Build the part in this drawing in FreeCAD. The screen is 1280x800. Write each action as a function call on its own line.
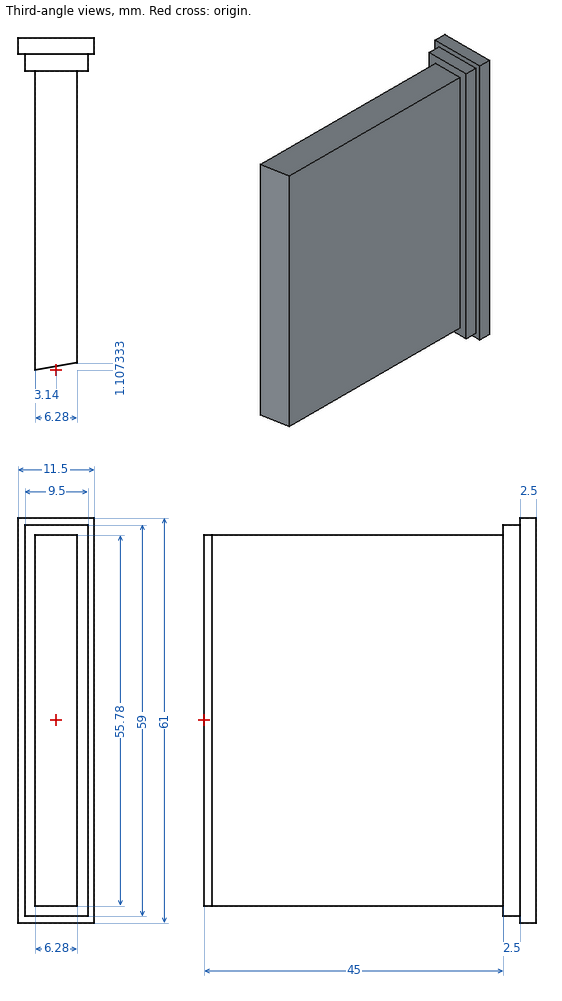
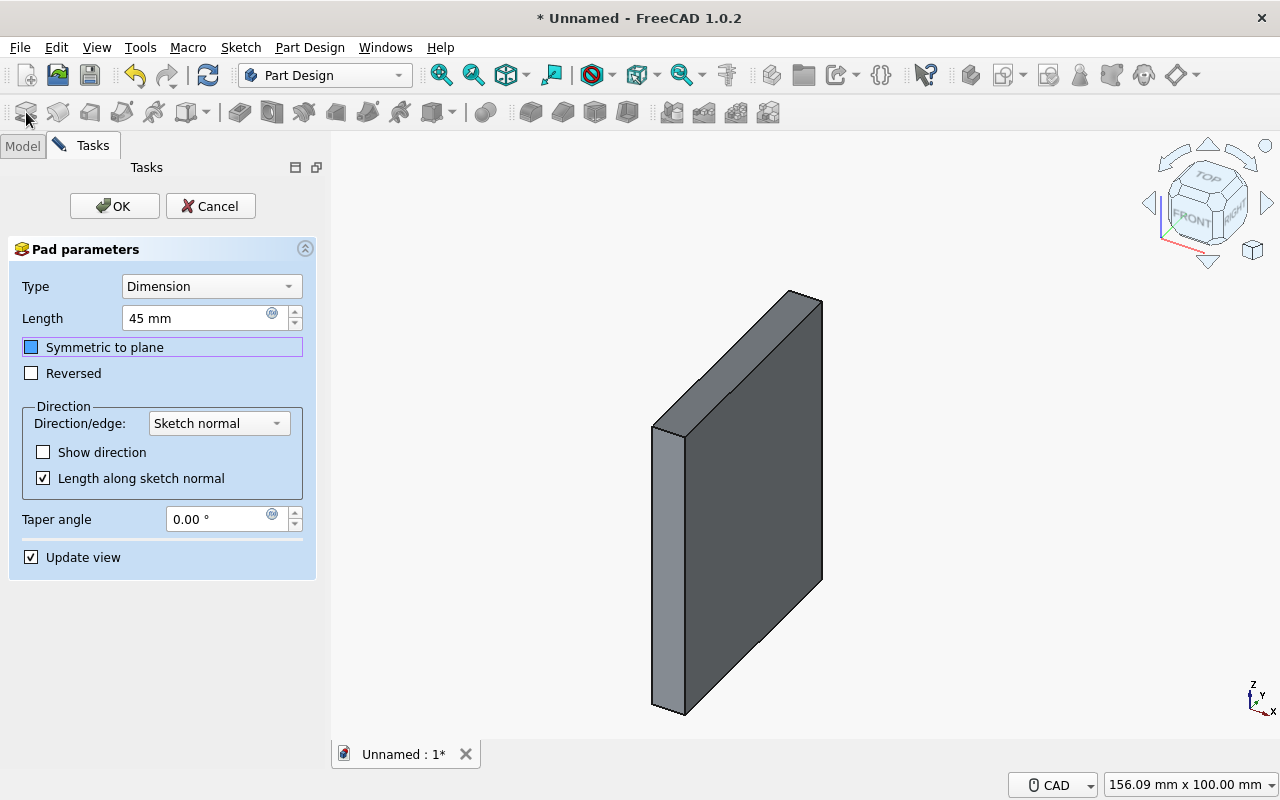
click(30, 373)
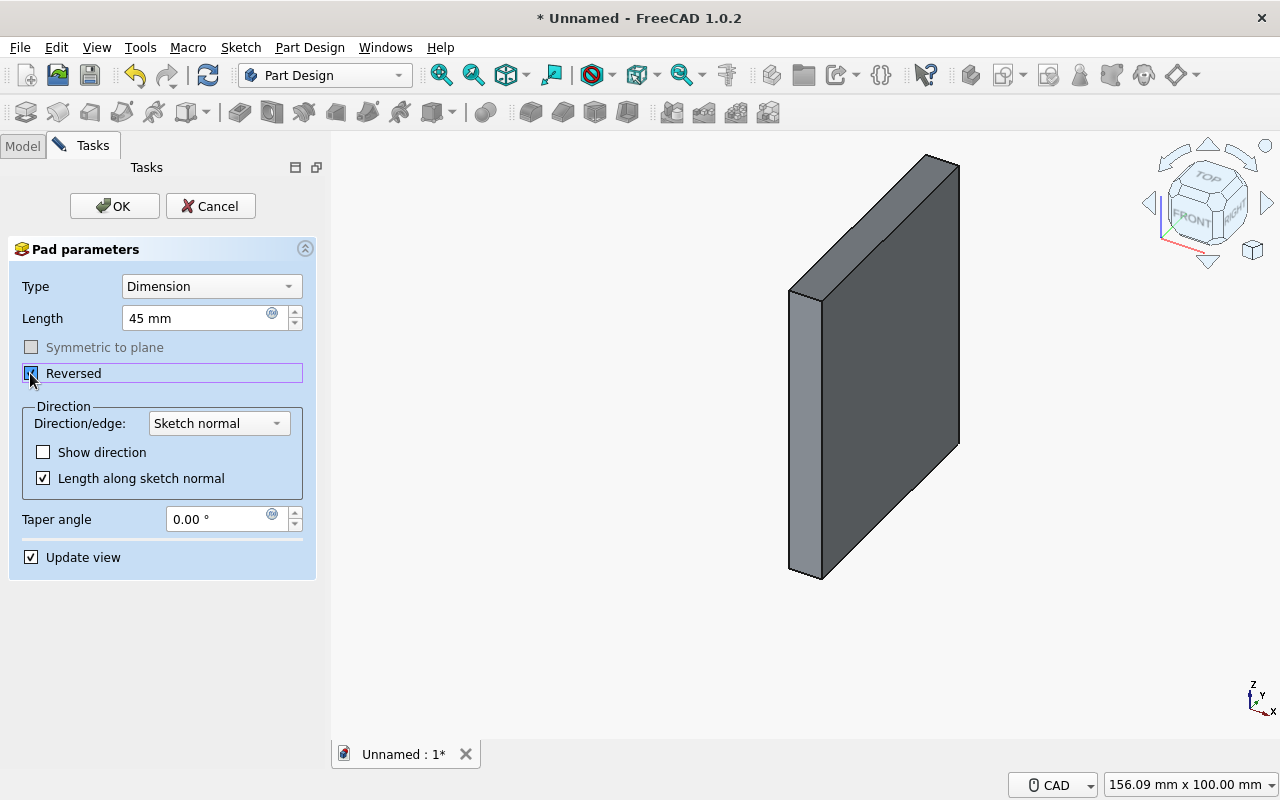
click(115, 206)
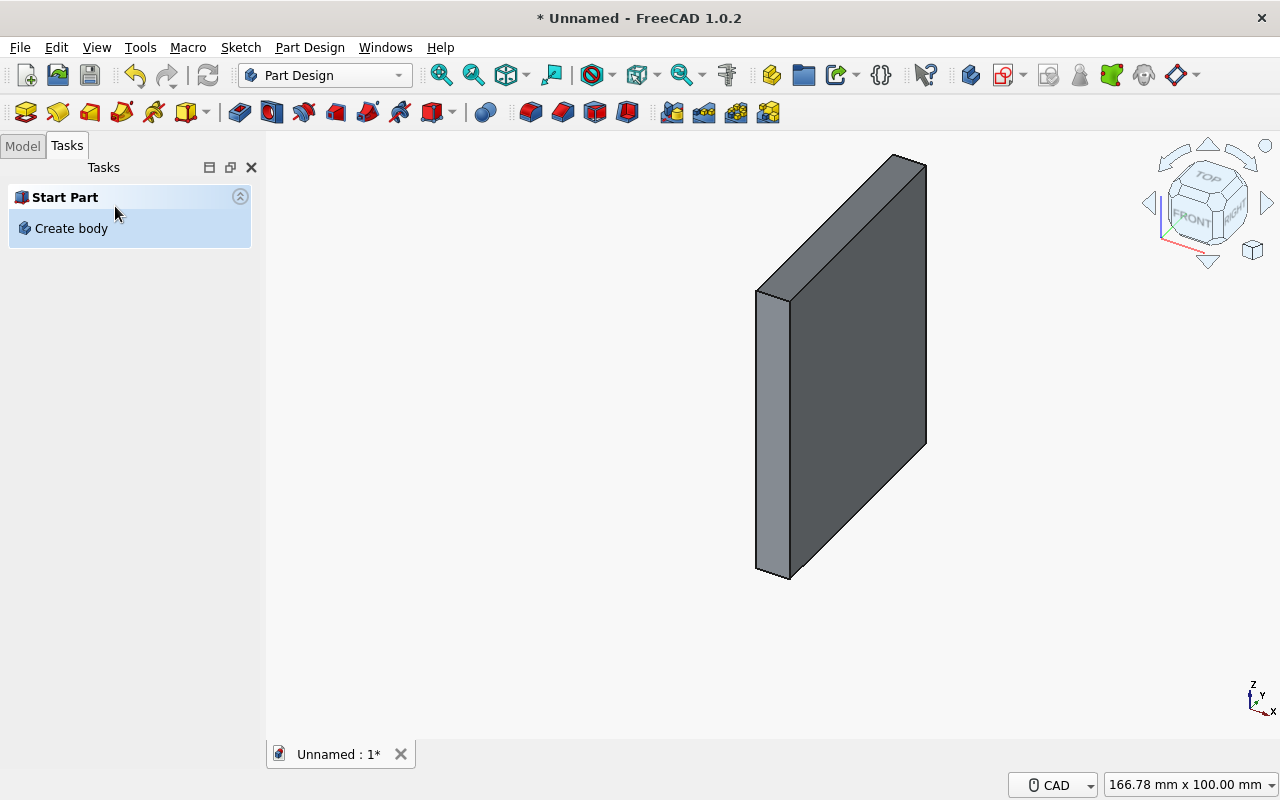
click(900, 169)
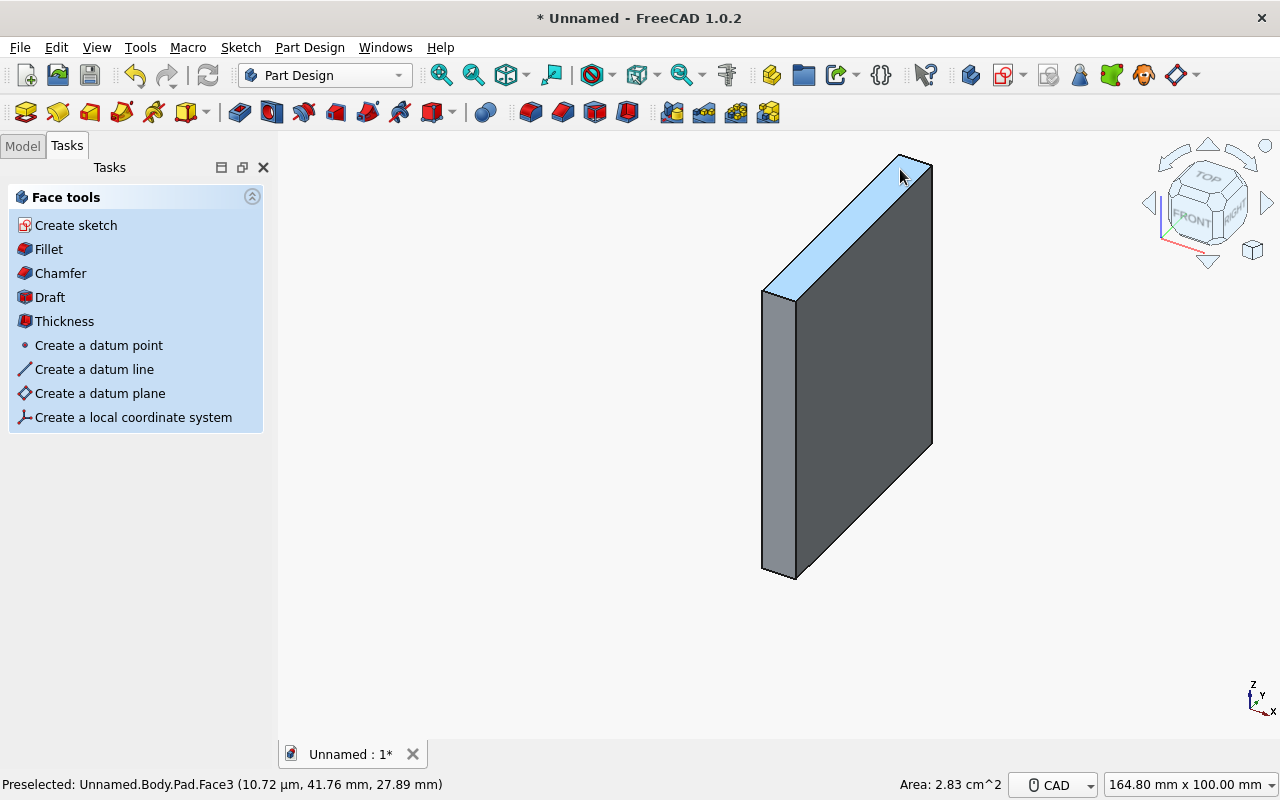
click(1004, 76)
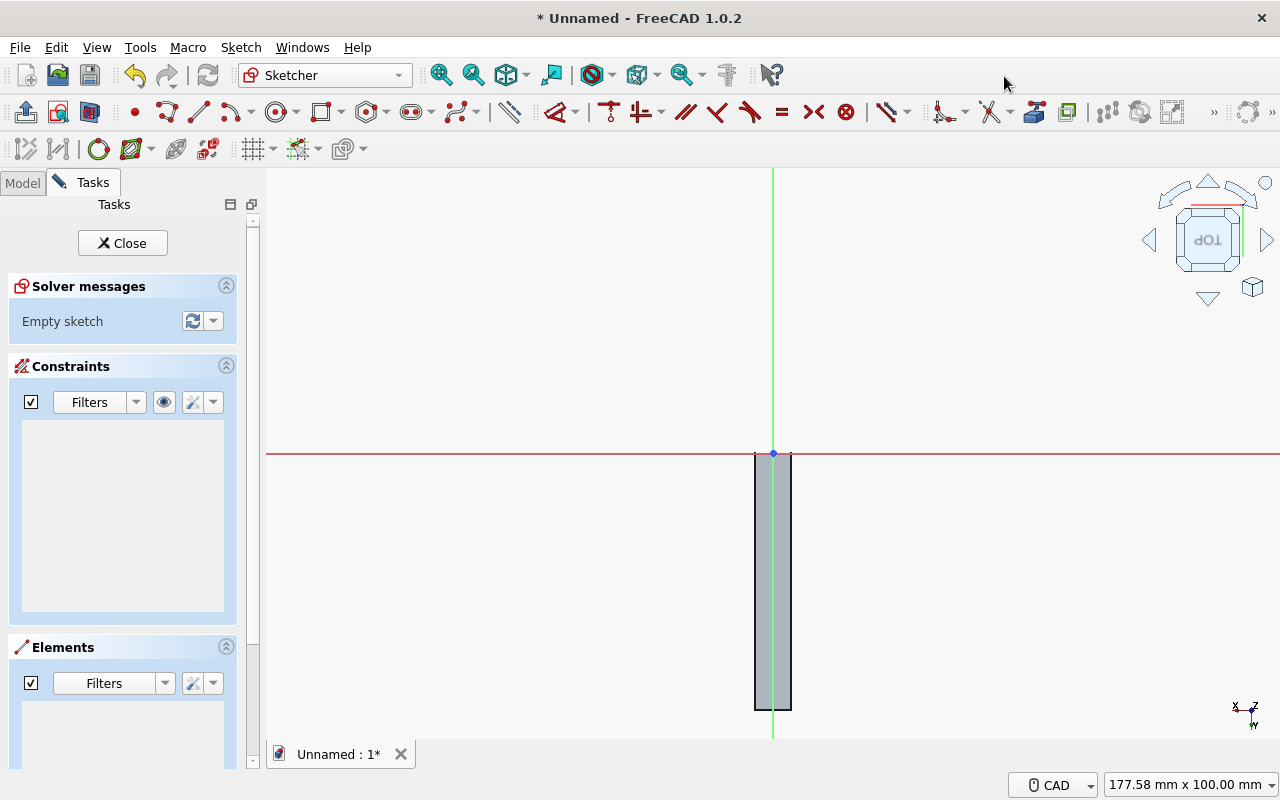
scroll(777, 457, up, 14)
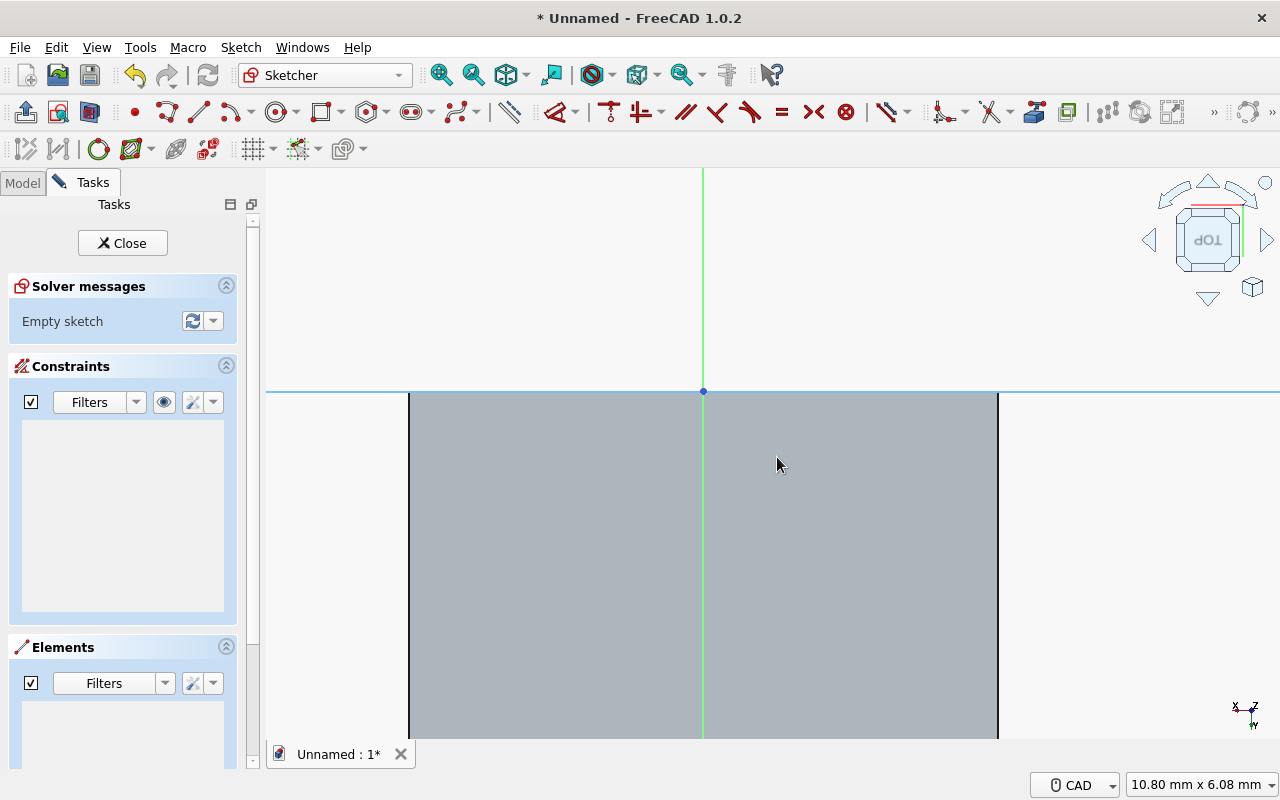
click(168, 112)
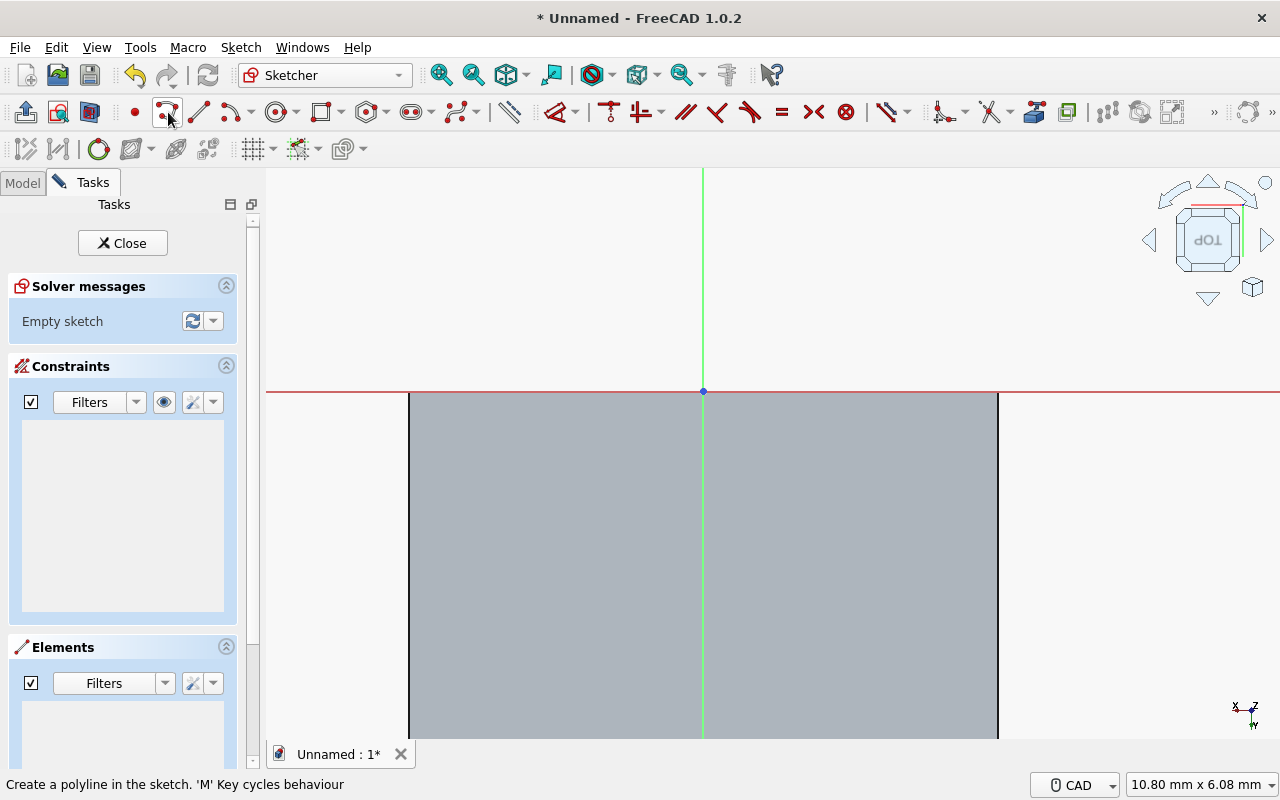
click(998, 392)
click(409, 401)
click(409, 496)
click(998, 392)
key(Escape)
key(Escape)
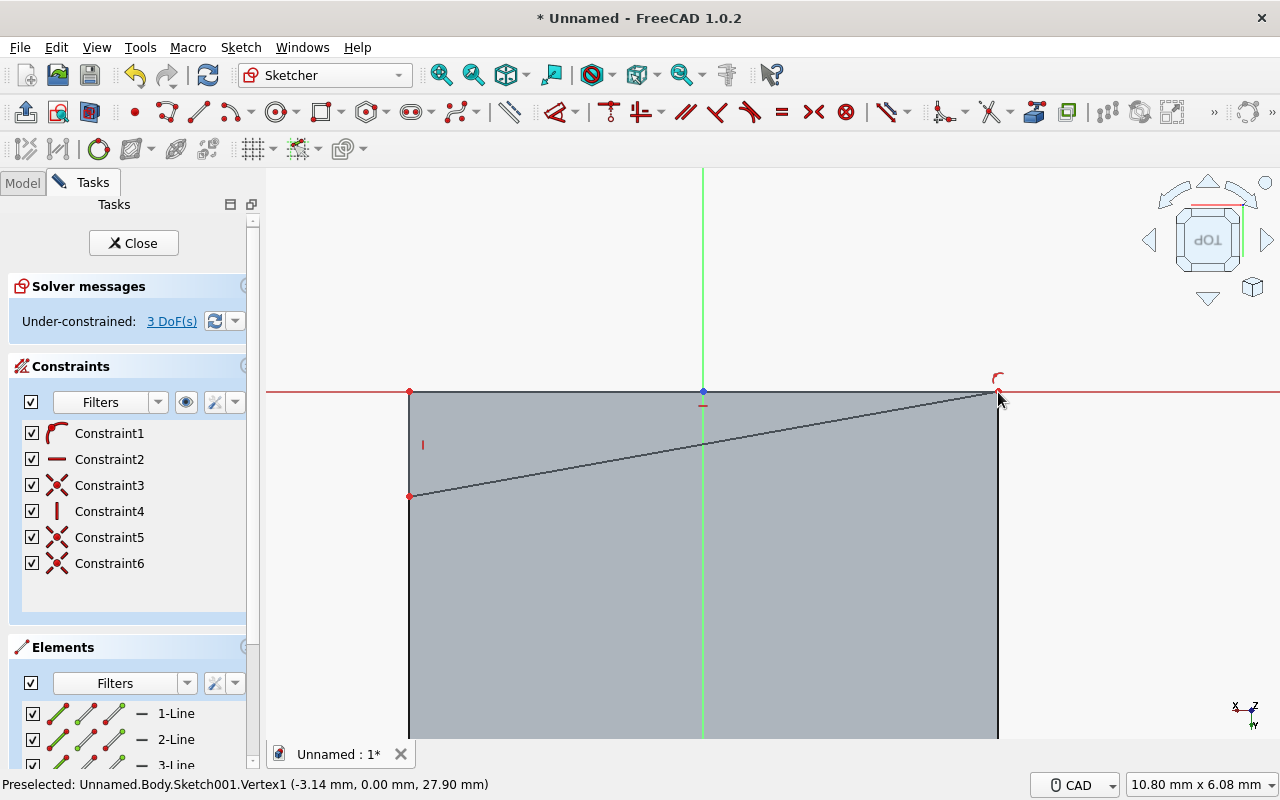
click(556, 112)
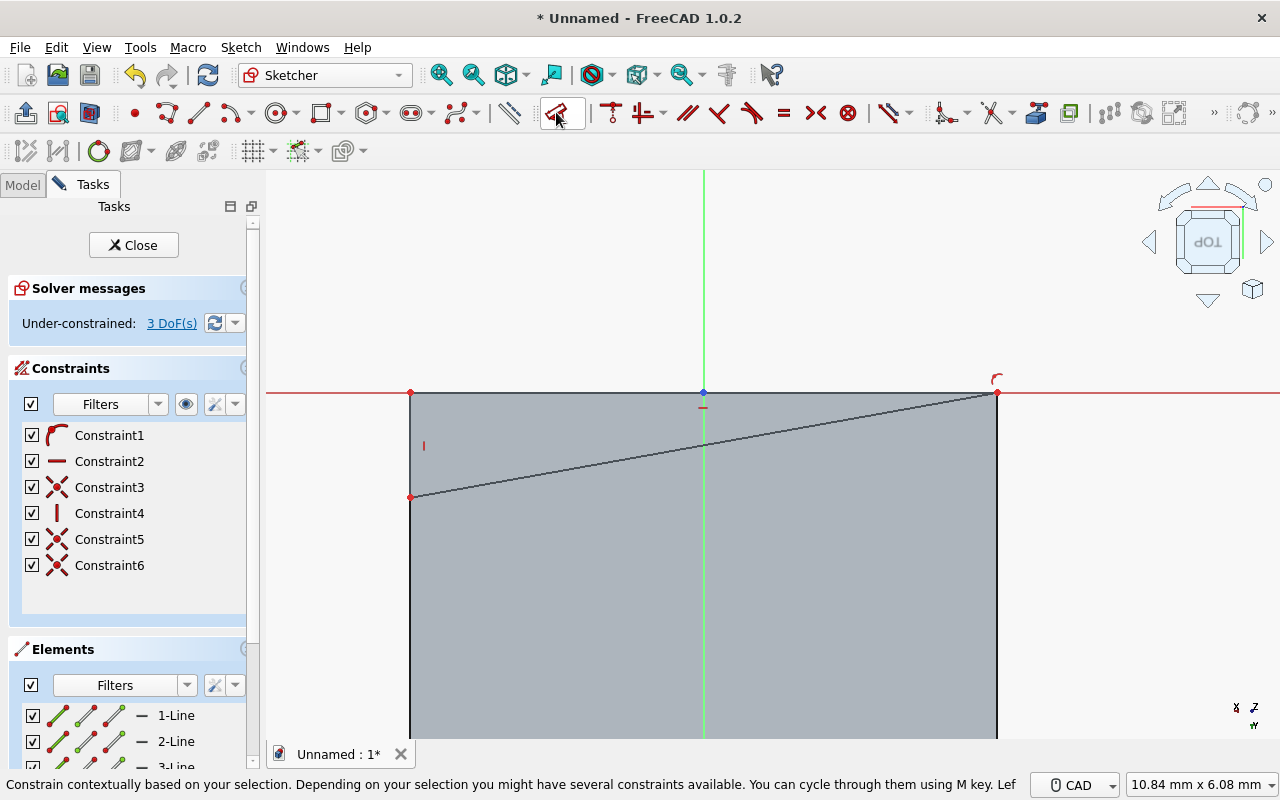
click(821, 393)
click(569, 359)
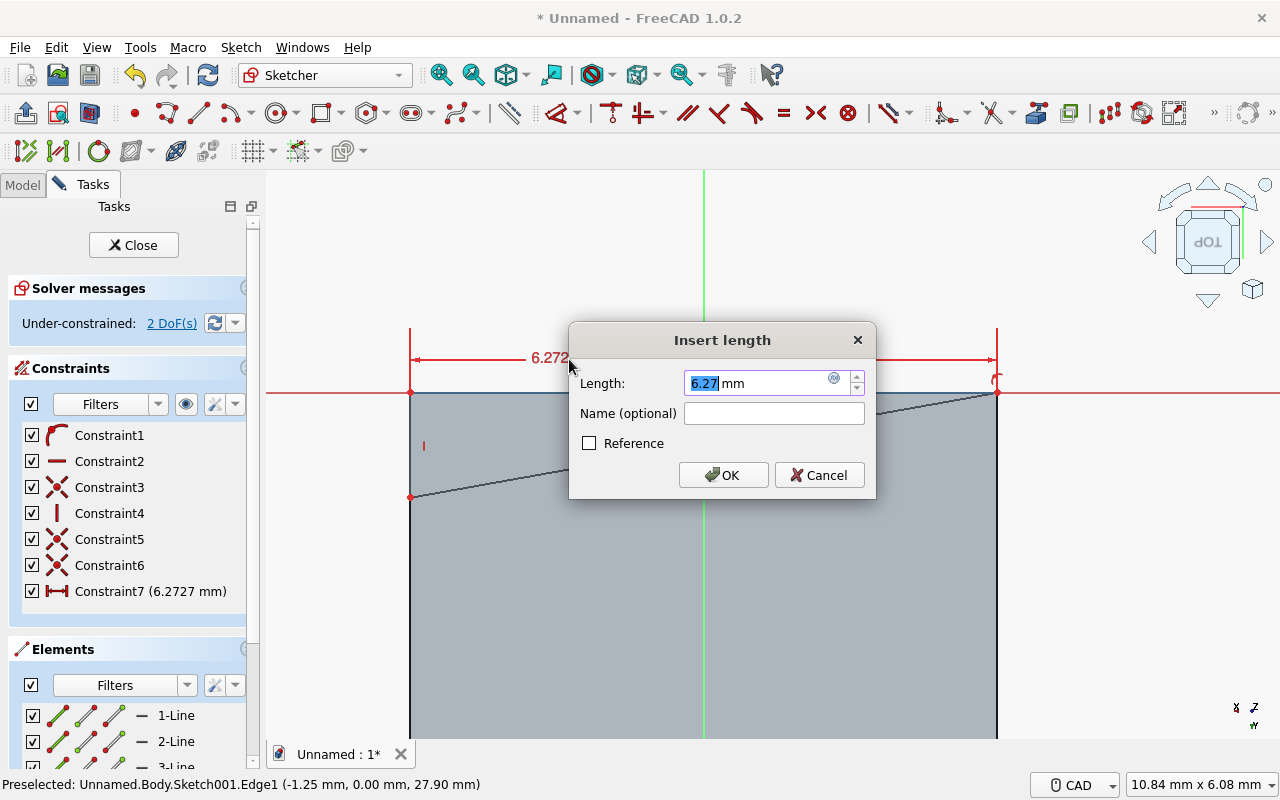
text(6.28)
key(Return)